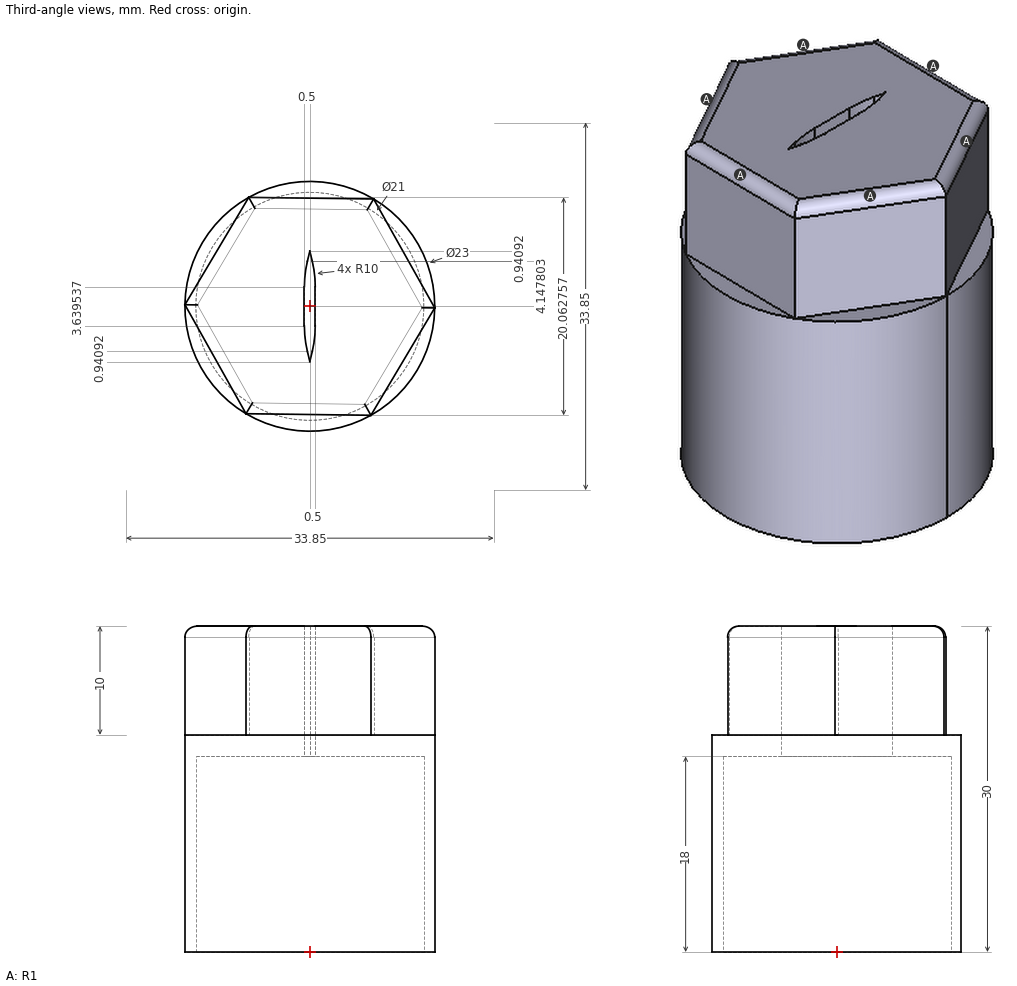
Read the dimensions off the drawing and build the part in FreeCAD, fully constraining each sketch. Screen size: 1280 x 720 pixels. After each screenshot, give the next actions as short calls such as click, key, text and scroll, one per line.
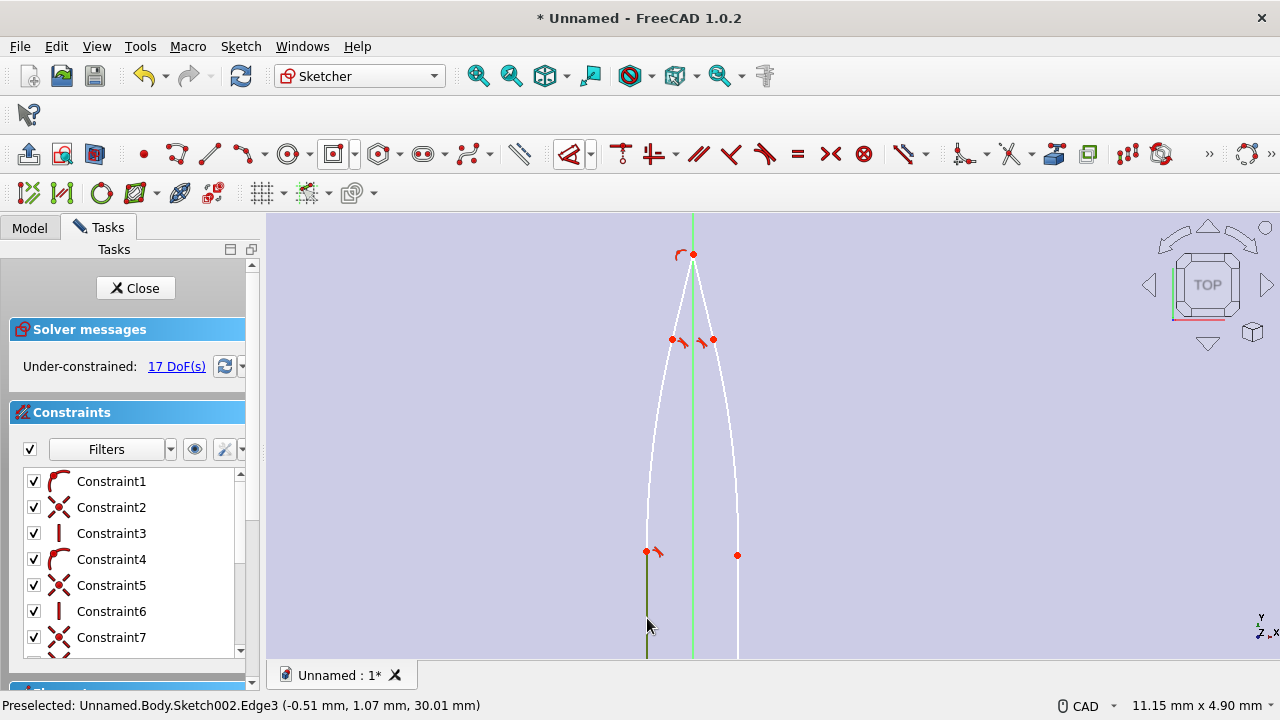
scroll(709, 315, down, 6)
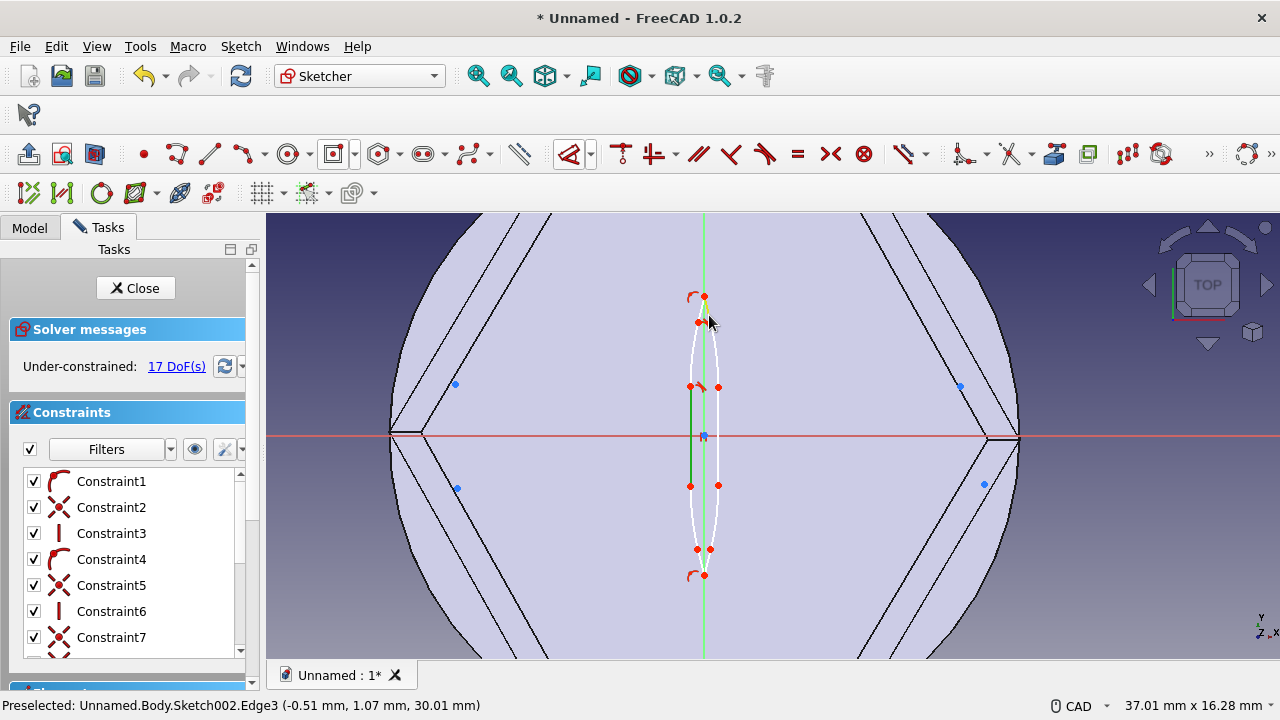
click(691, 506)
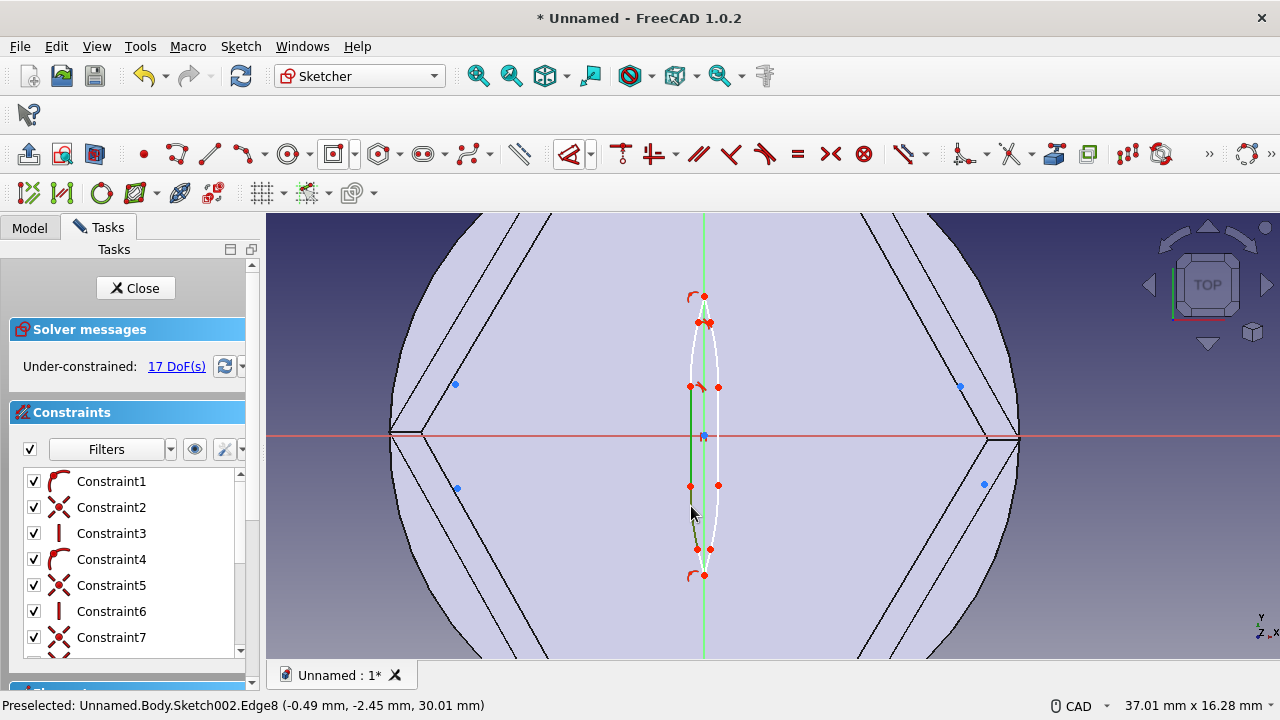
click(765, 154)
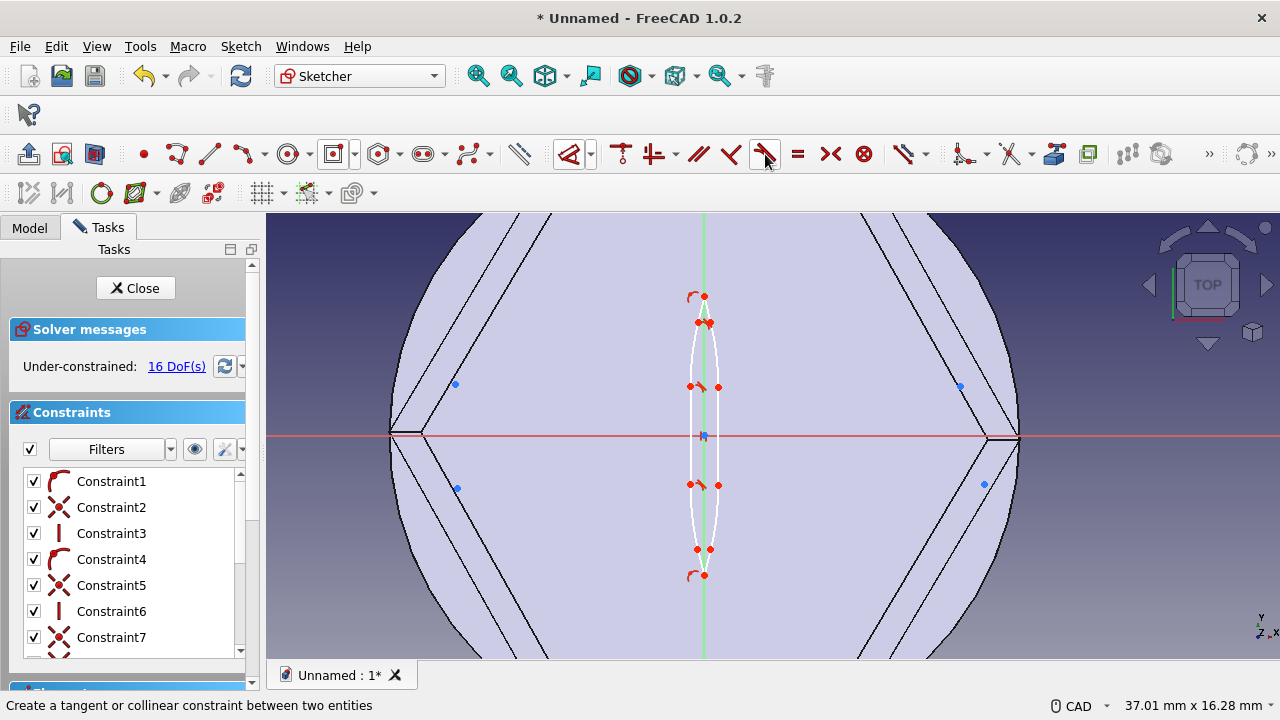
scroll(701, 560, up, 4)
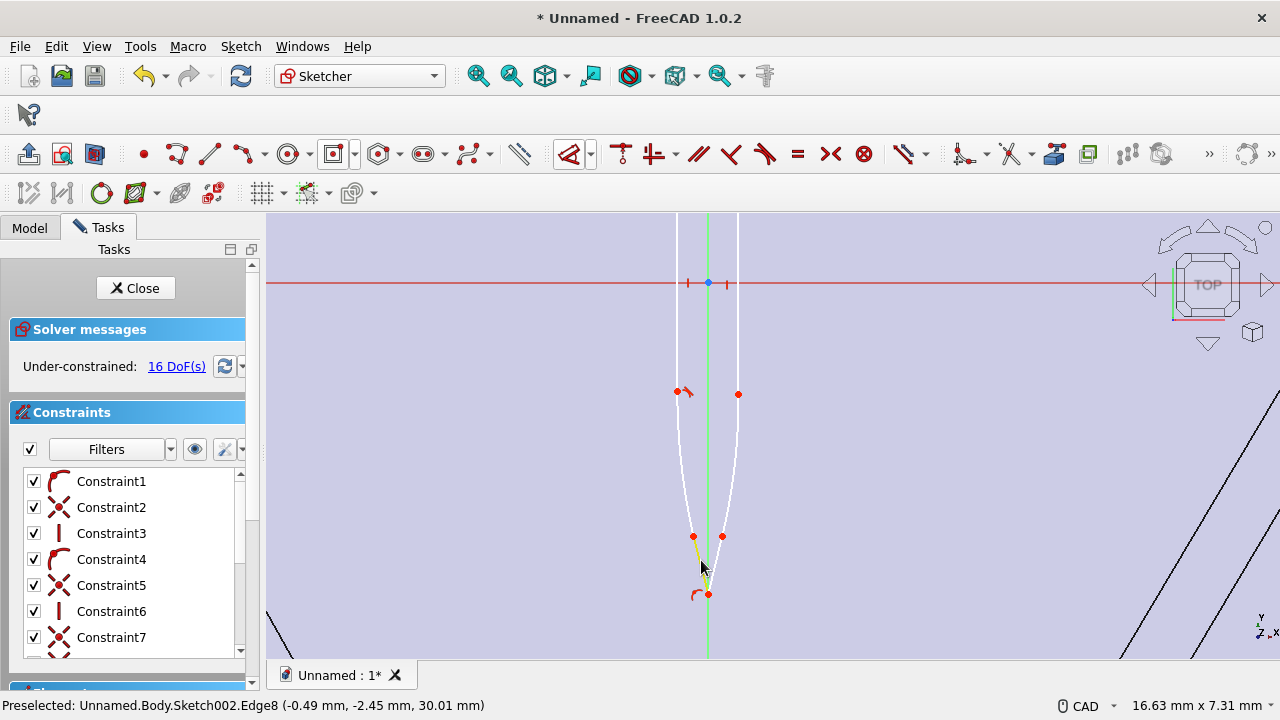
click(699, 560)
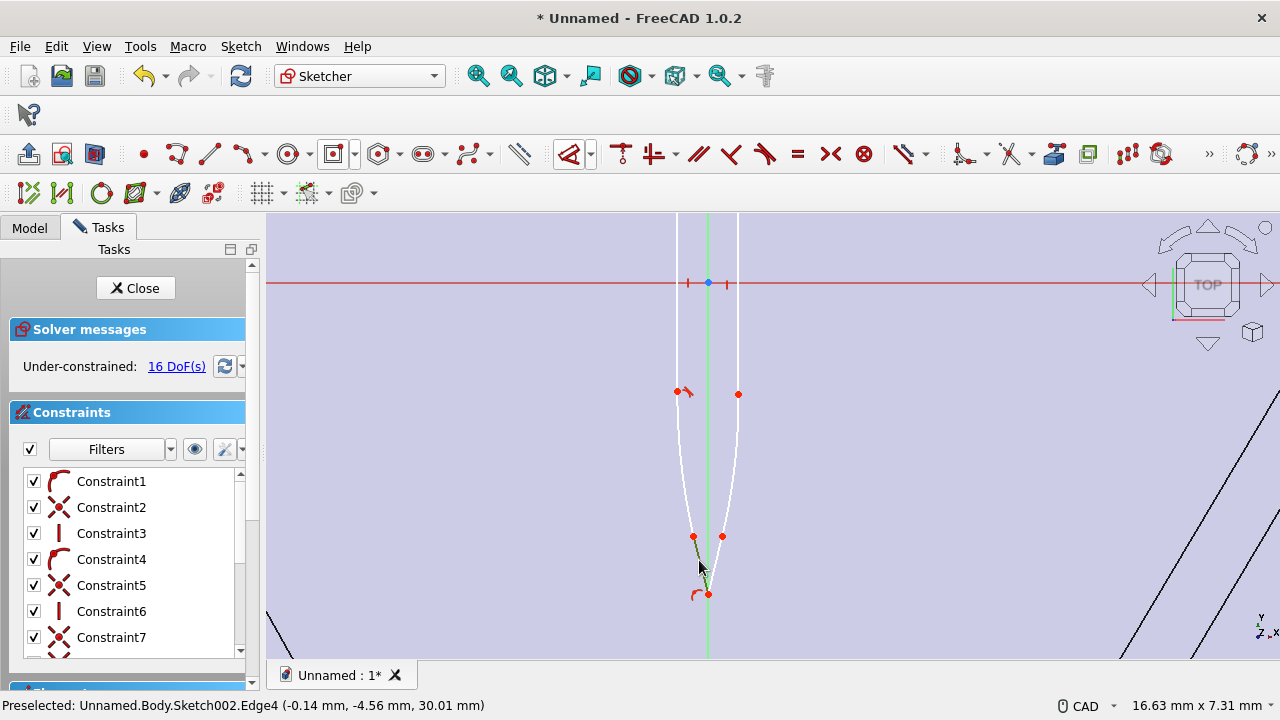
click(679, 436)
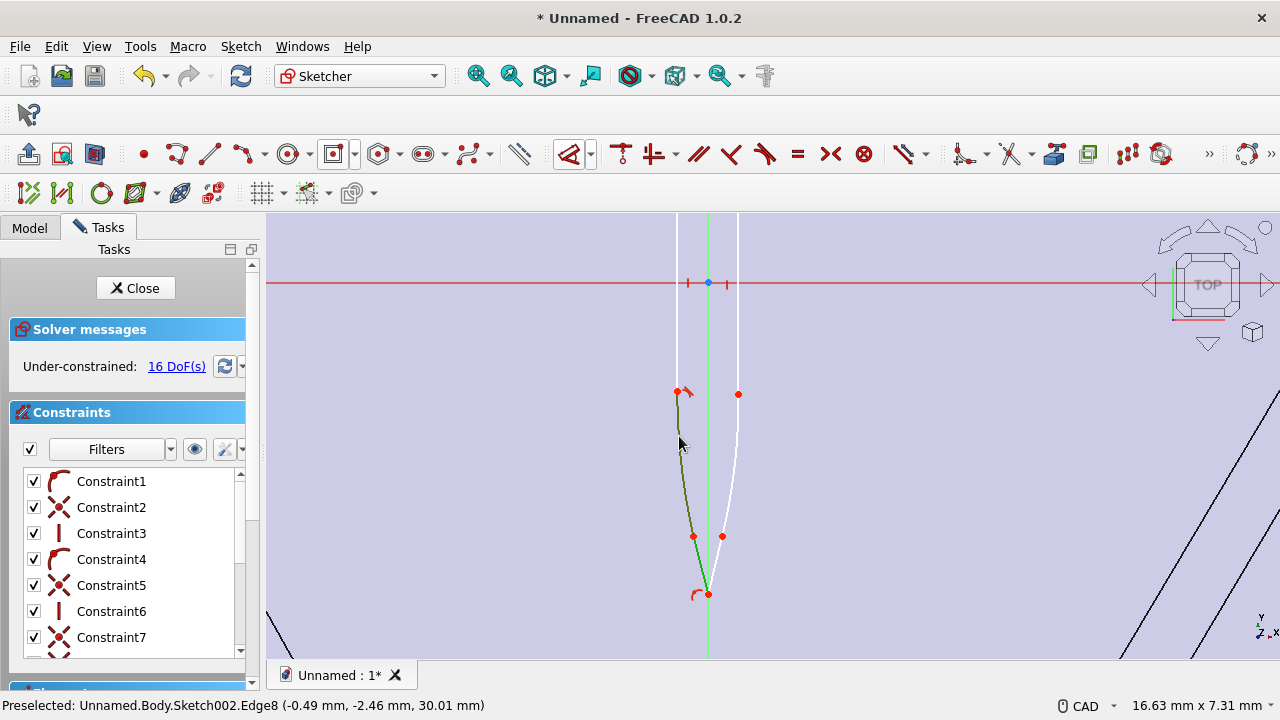
click(765, 154)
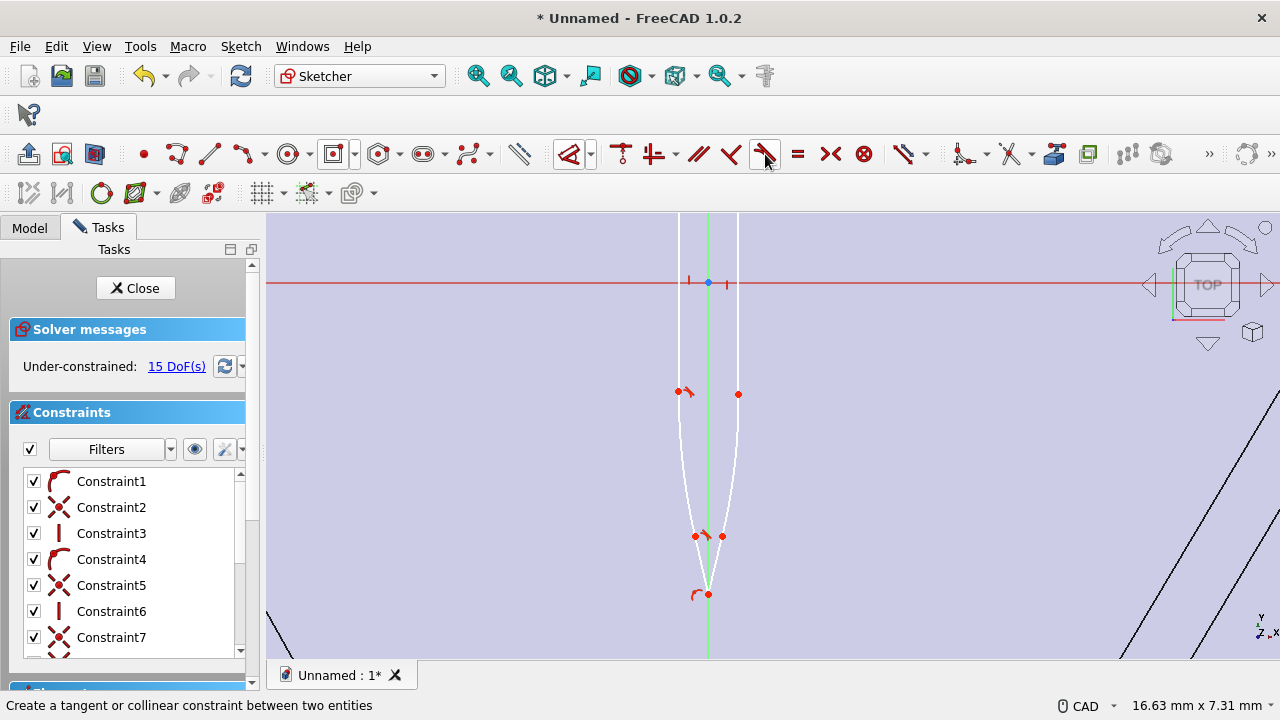
scroll(718, 554, up, 2)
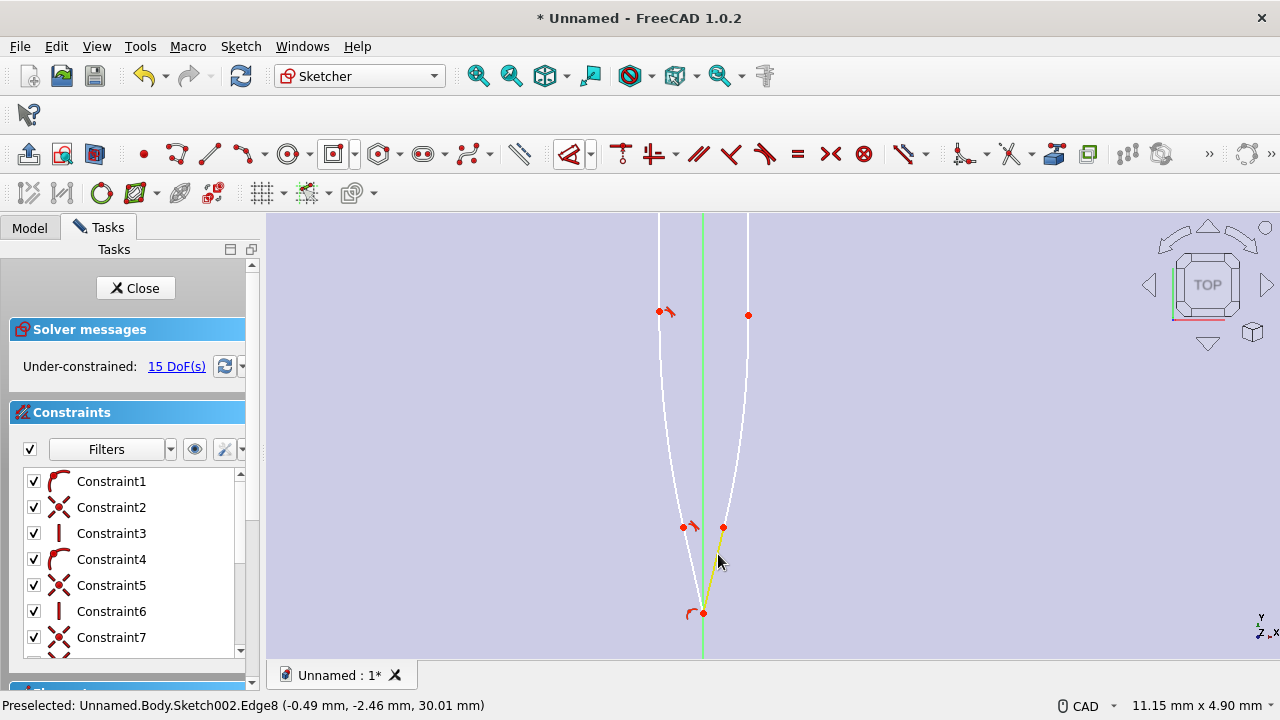
click(718, 554)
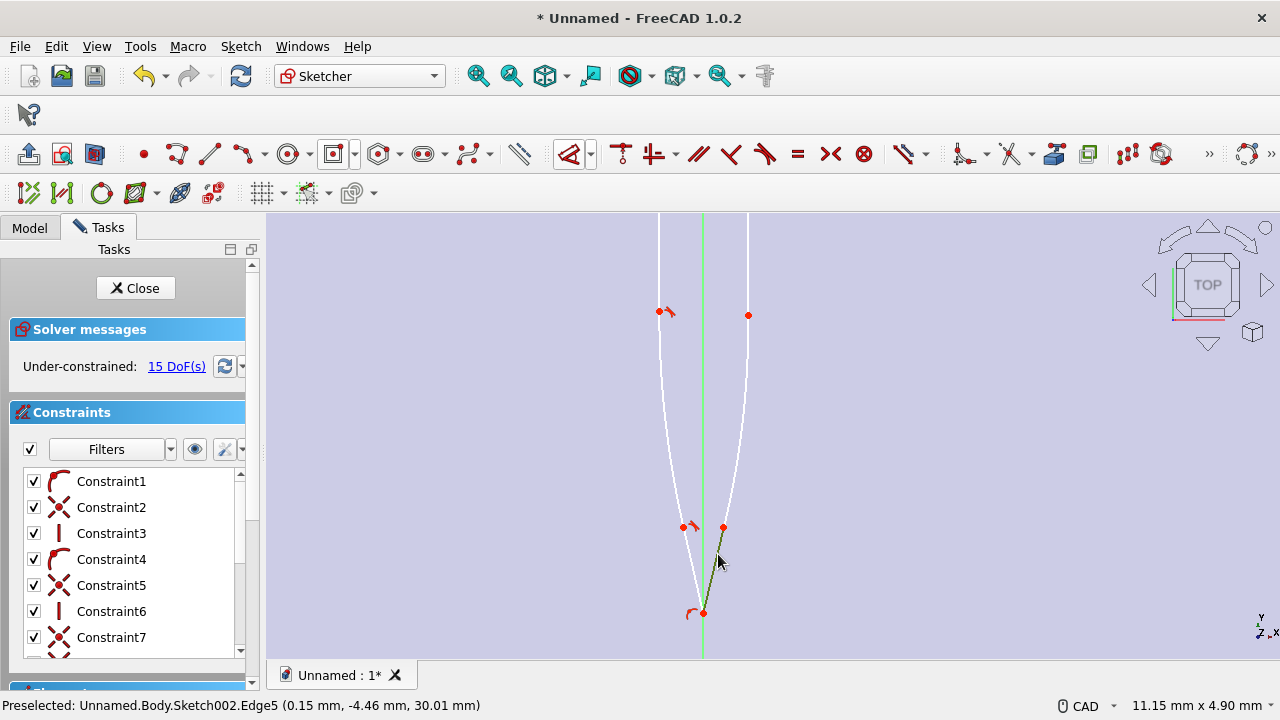
click(737, 465)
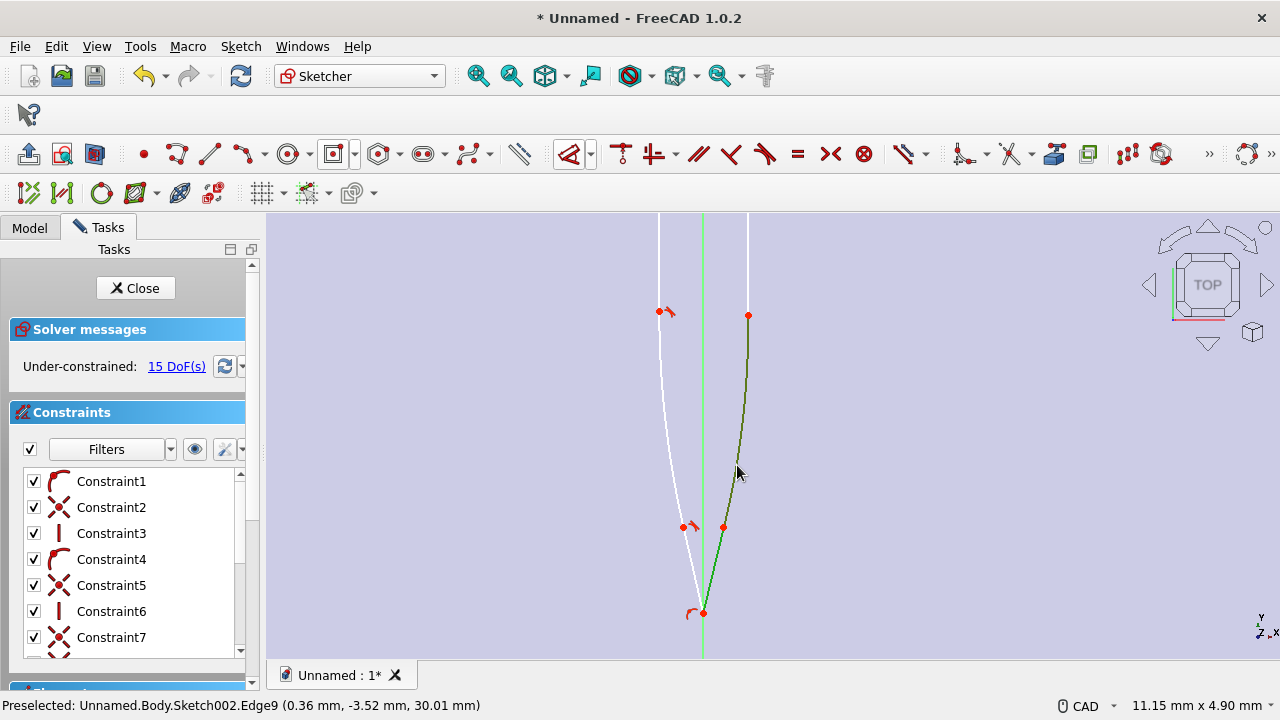
key(t)